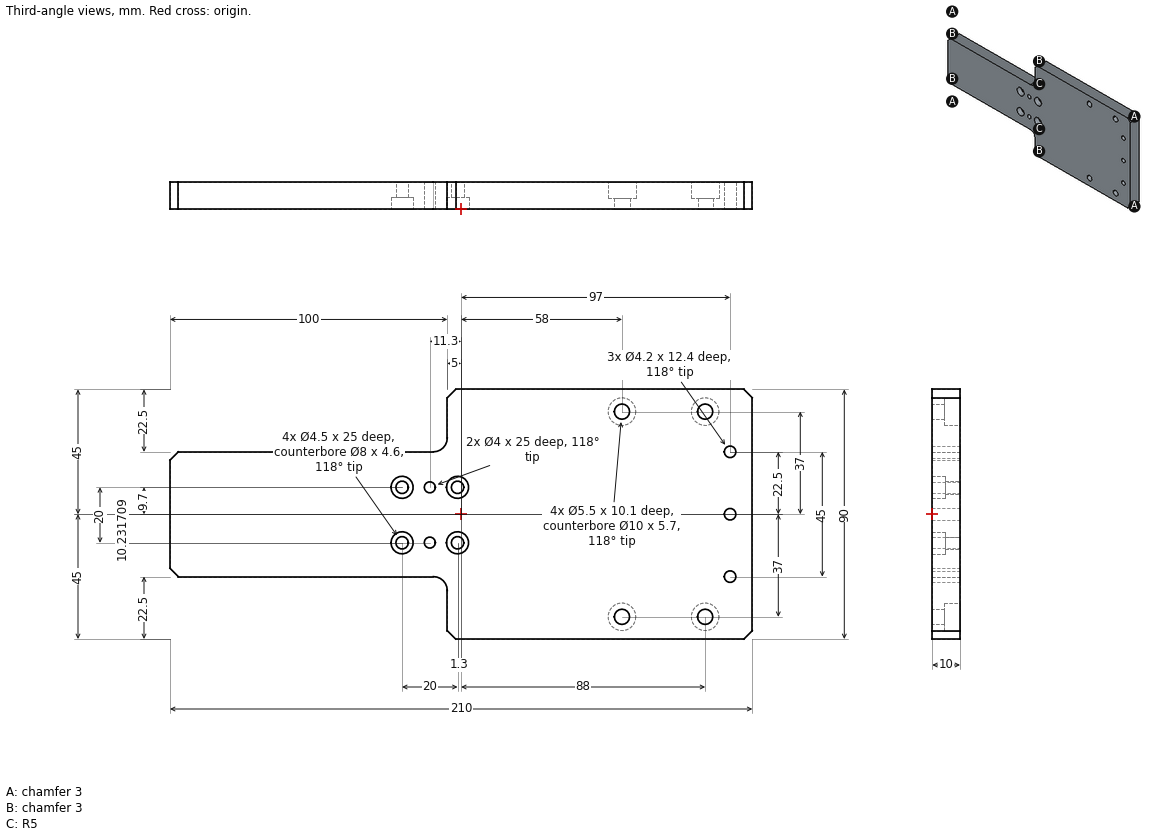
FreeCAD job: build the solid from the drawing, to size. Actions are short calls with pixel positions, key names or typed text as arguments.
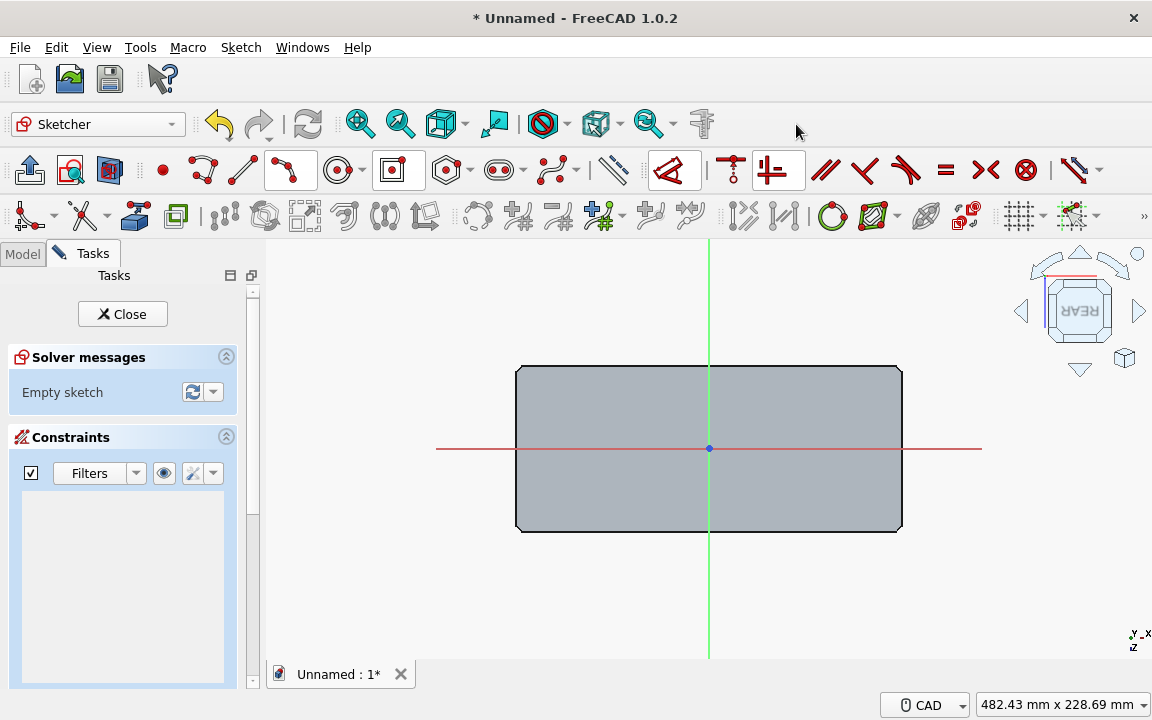
scroll(977, 449, up, 3)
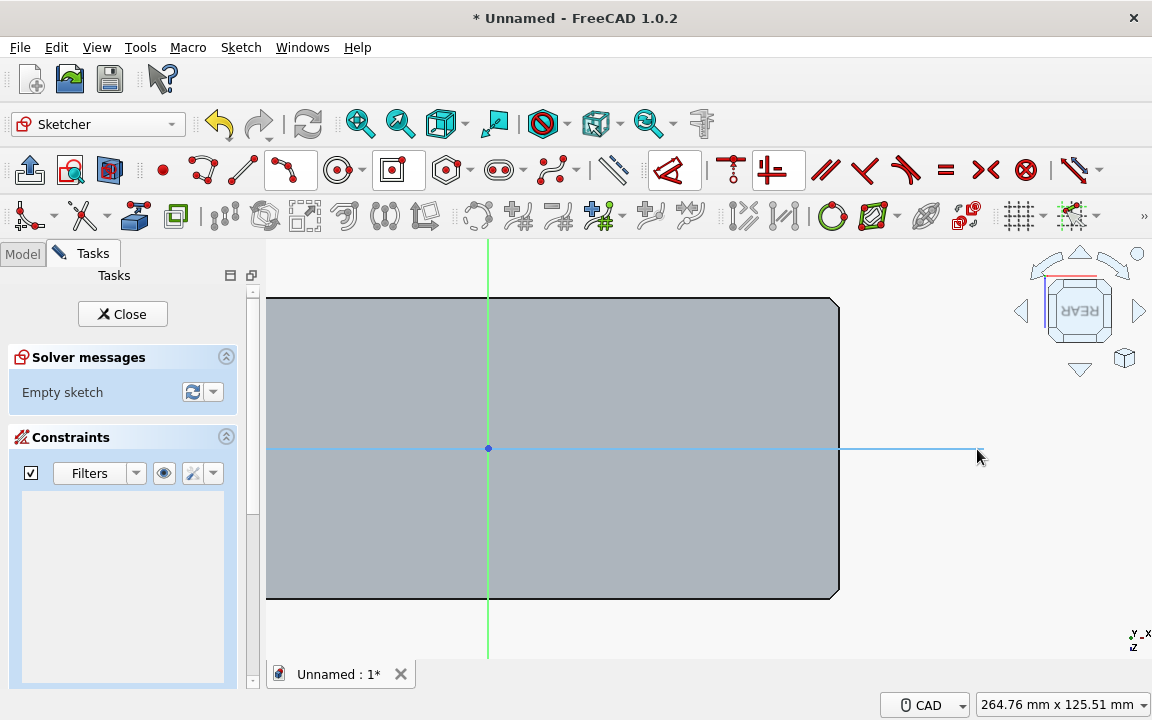
click(338, 170)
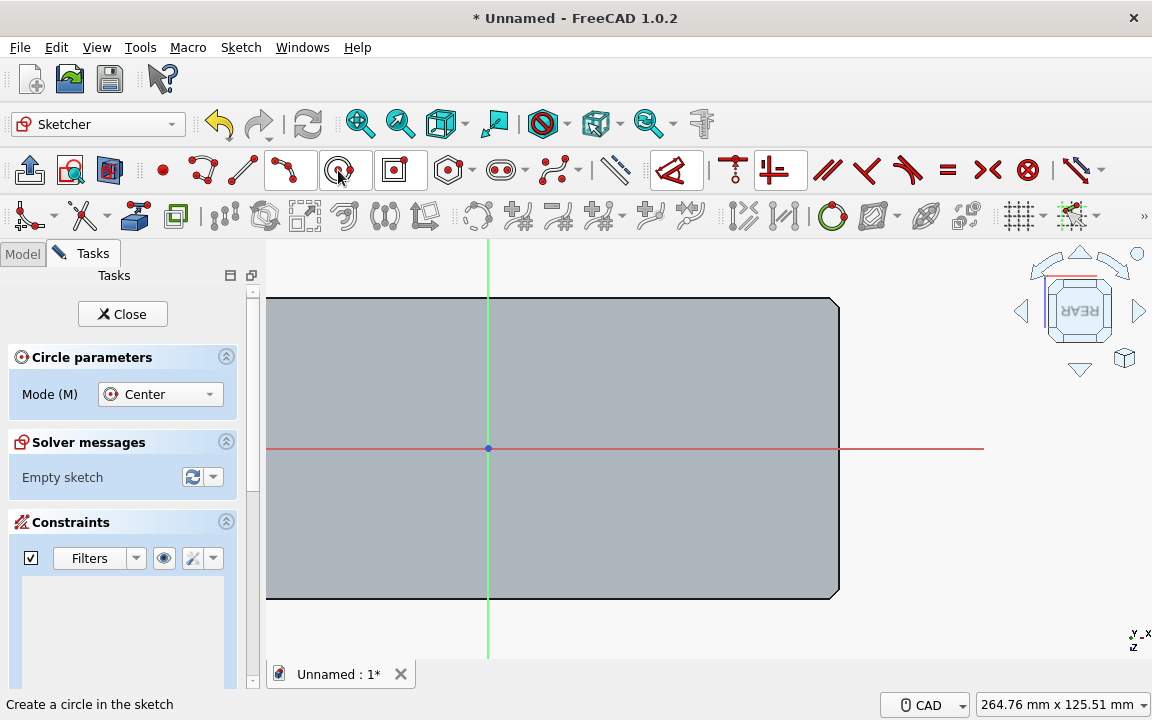
scroll(682, 572, up, 5)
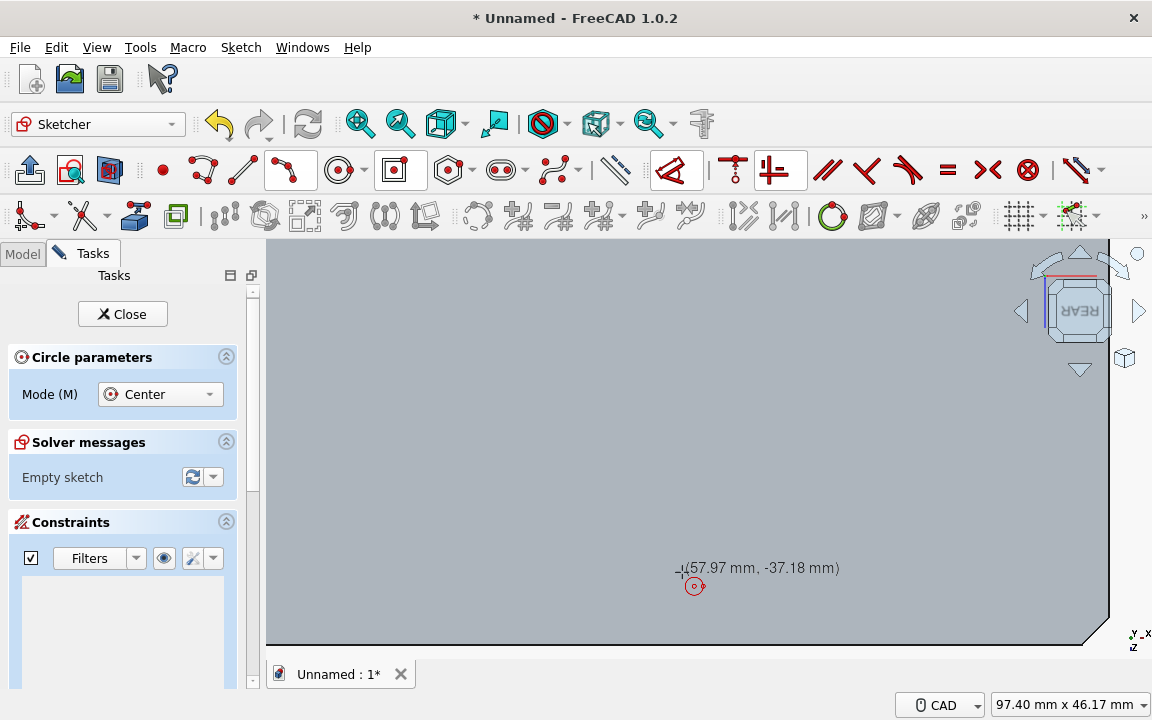
click(681, 572)
click(699, 554)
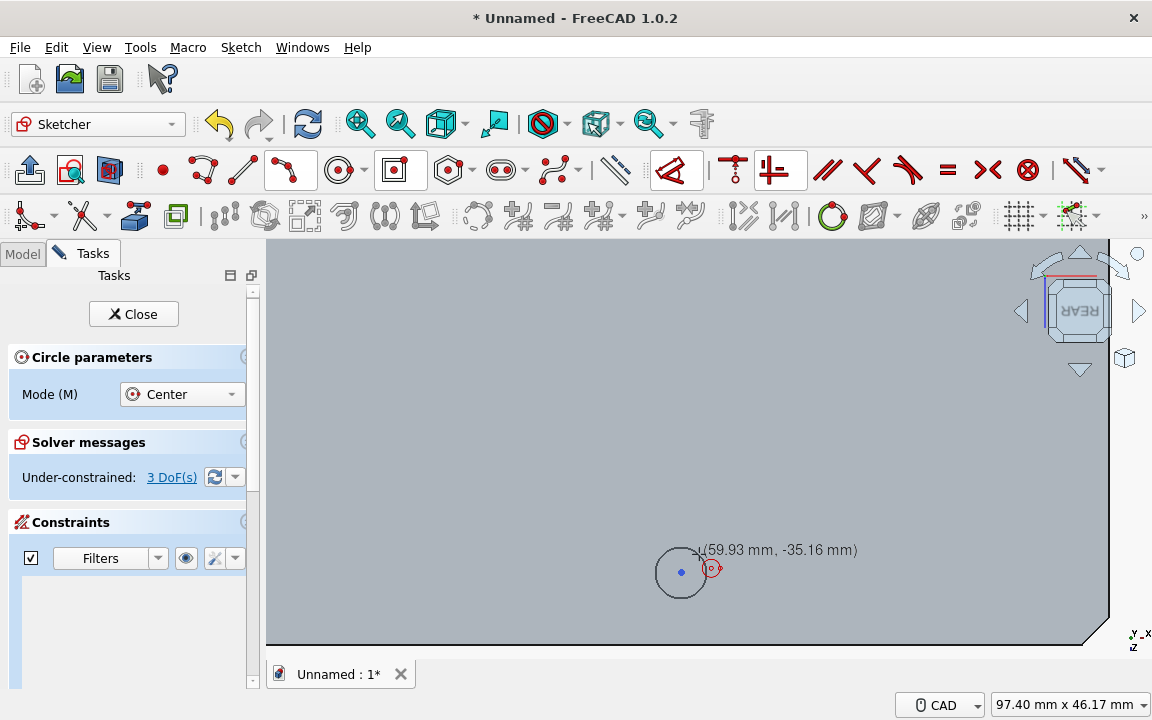
scroll(683, 573, down, 5)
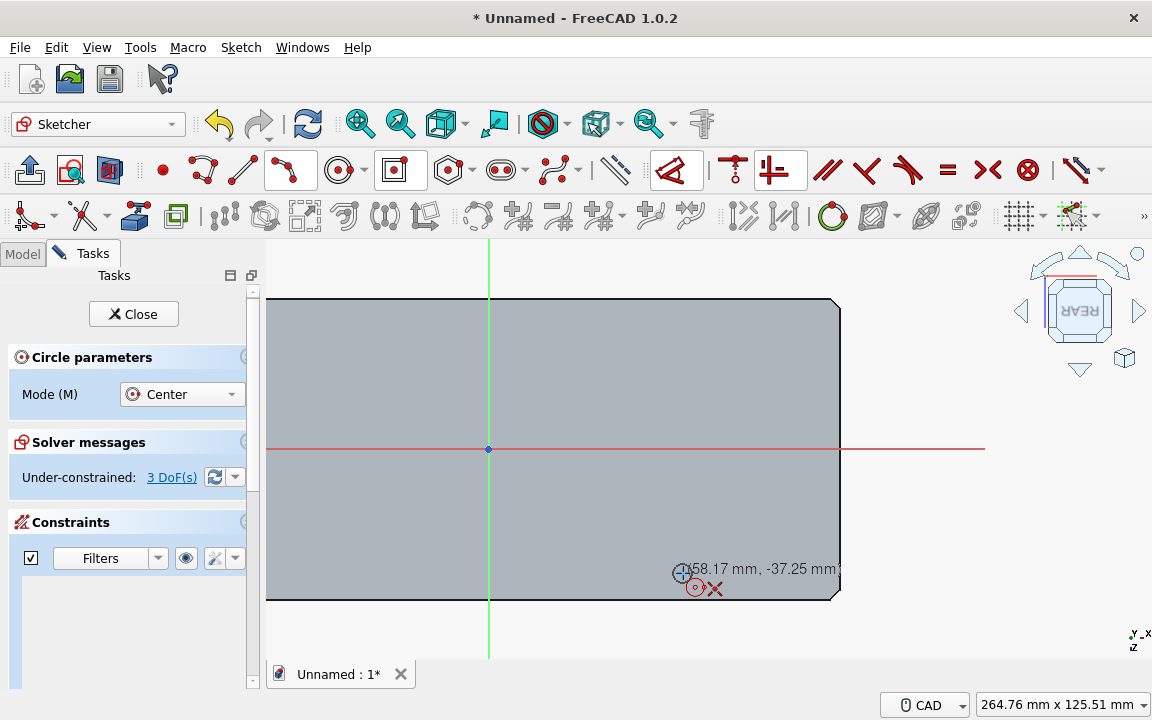
scroll(683, 325, up, 5)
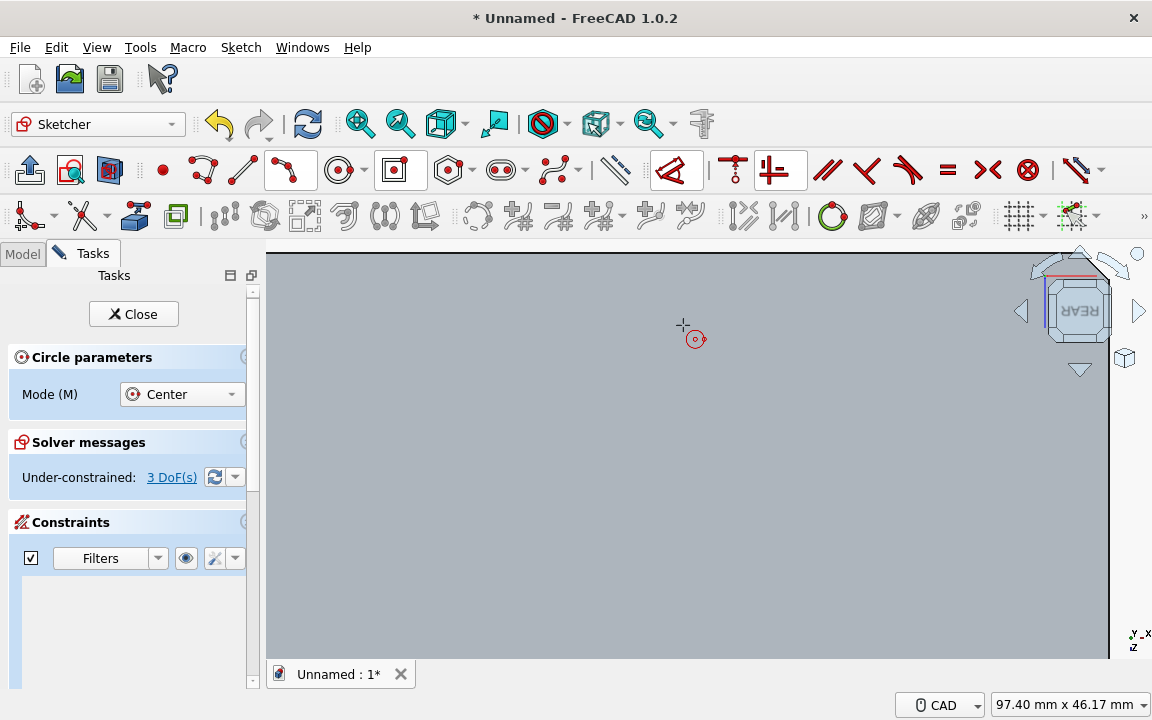
click(681, 326)
click(699, 308)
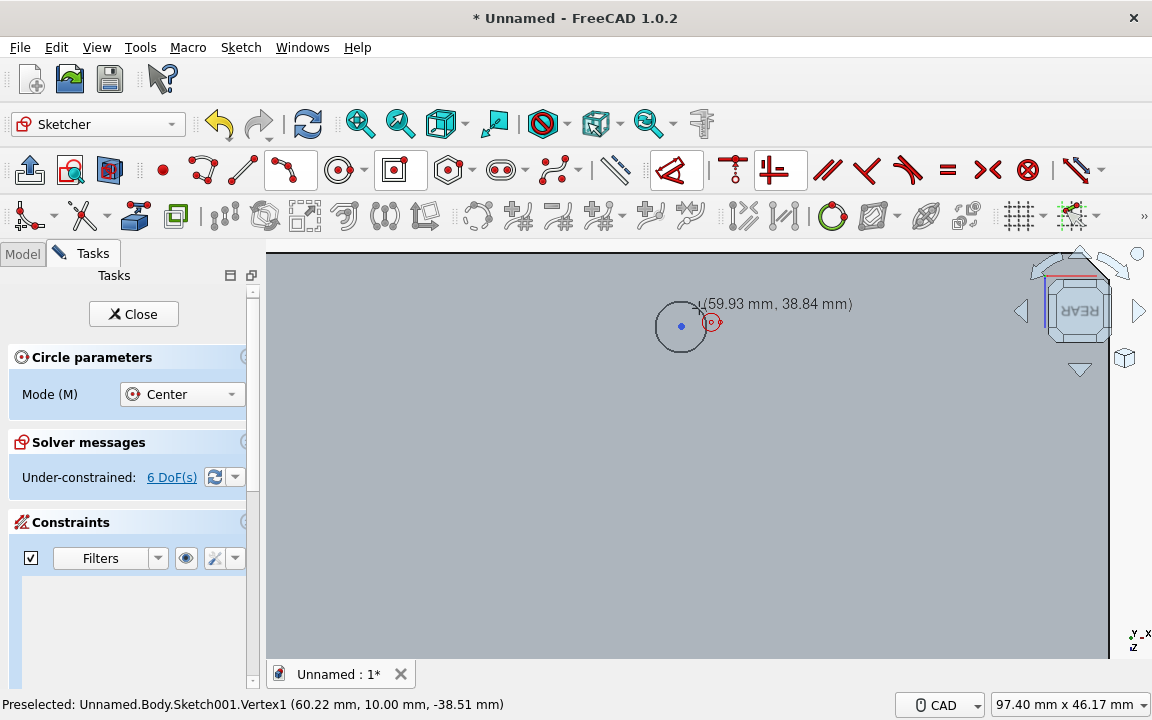
click(954, 326)
click(972, 308)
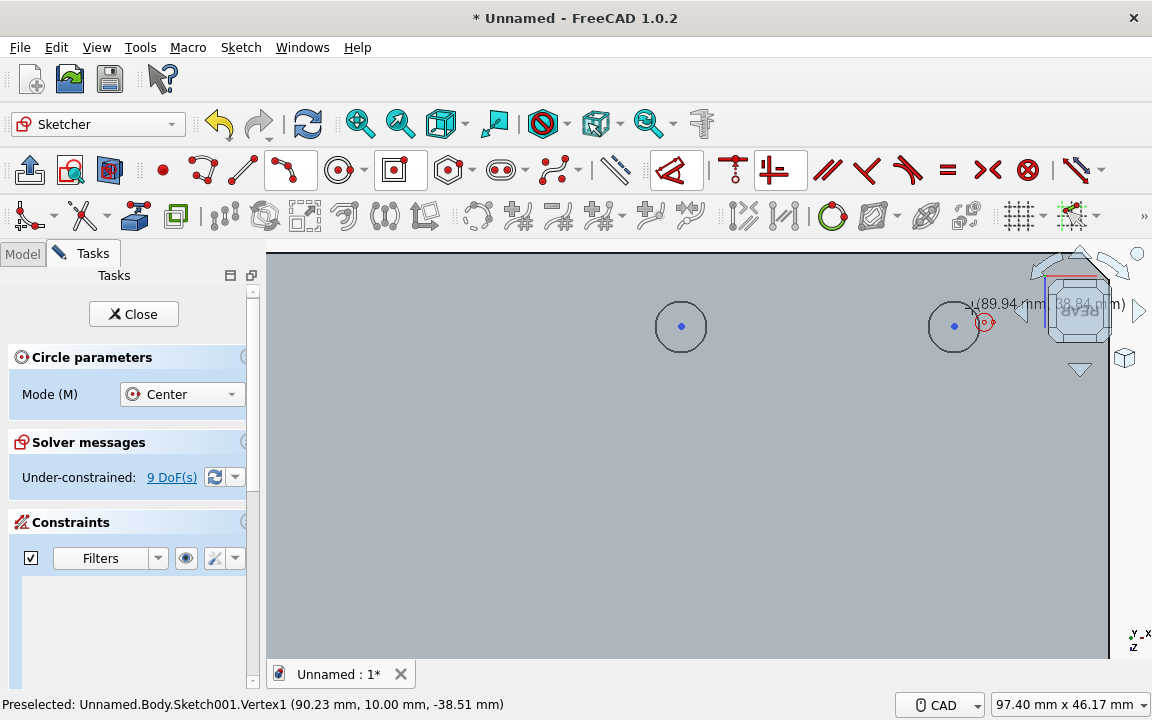
scroll(683, 325, down, 5)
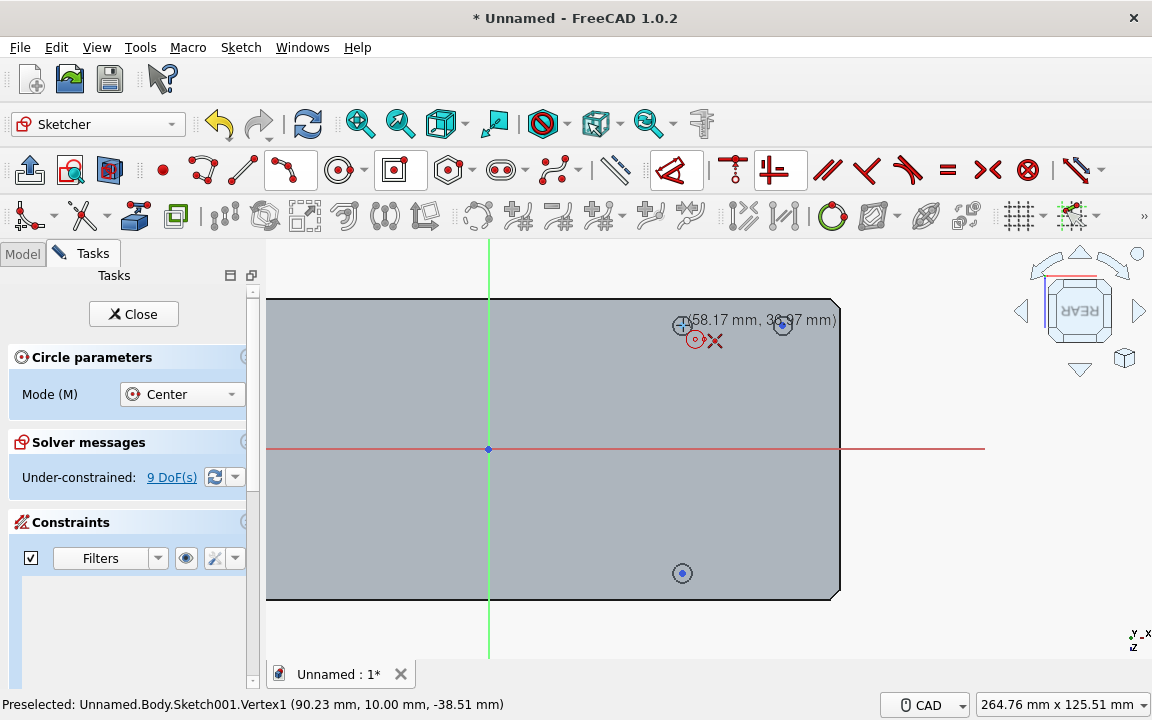
scroll(783, 573, up, 5)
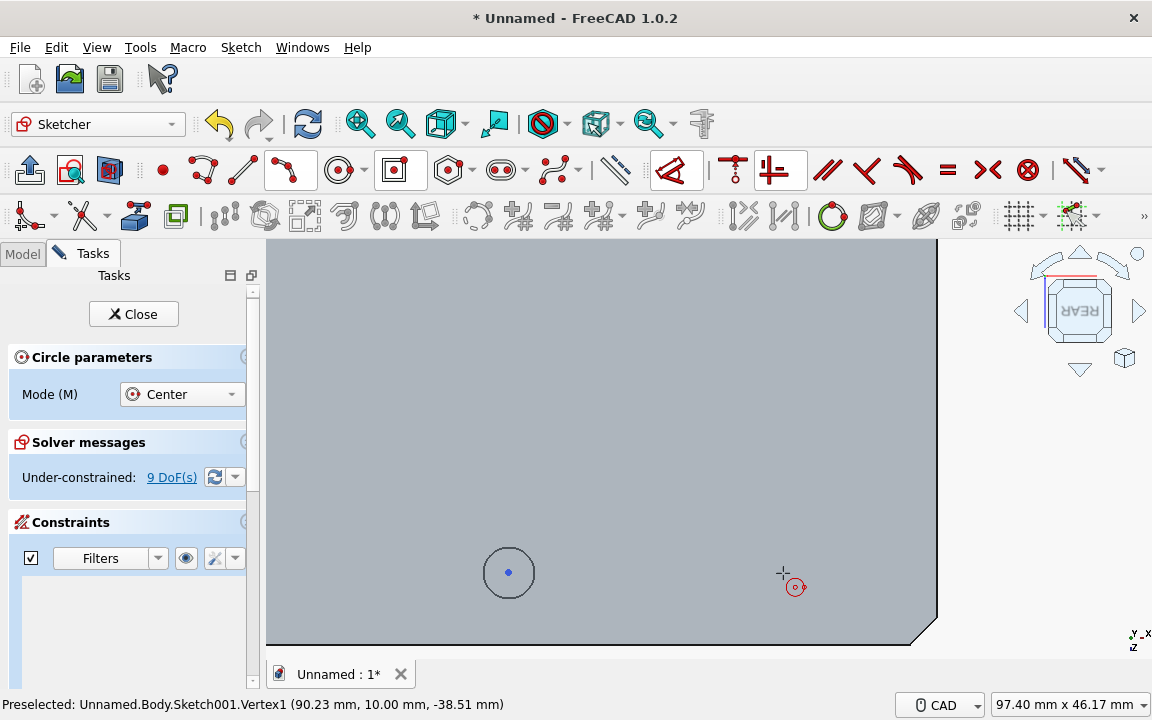
click(782, 572)
click(800, 554)
key(Escape)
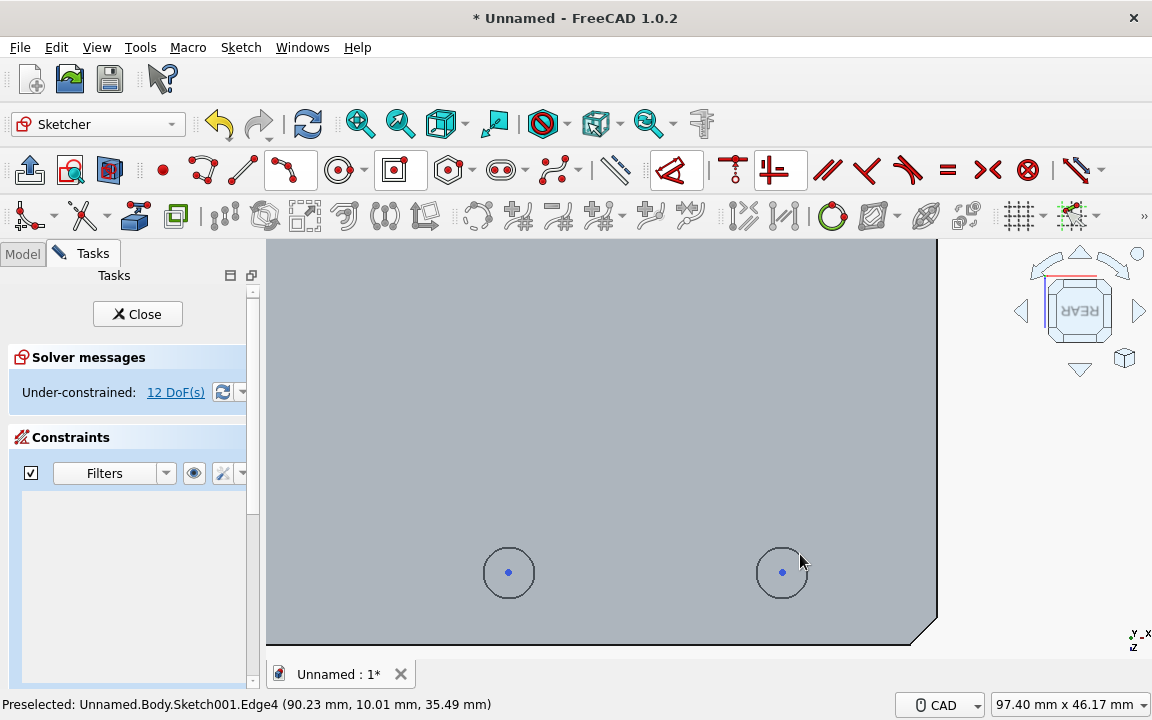
click(527, 555)